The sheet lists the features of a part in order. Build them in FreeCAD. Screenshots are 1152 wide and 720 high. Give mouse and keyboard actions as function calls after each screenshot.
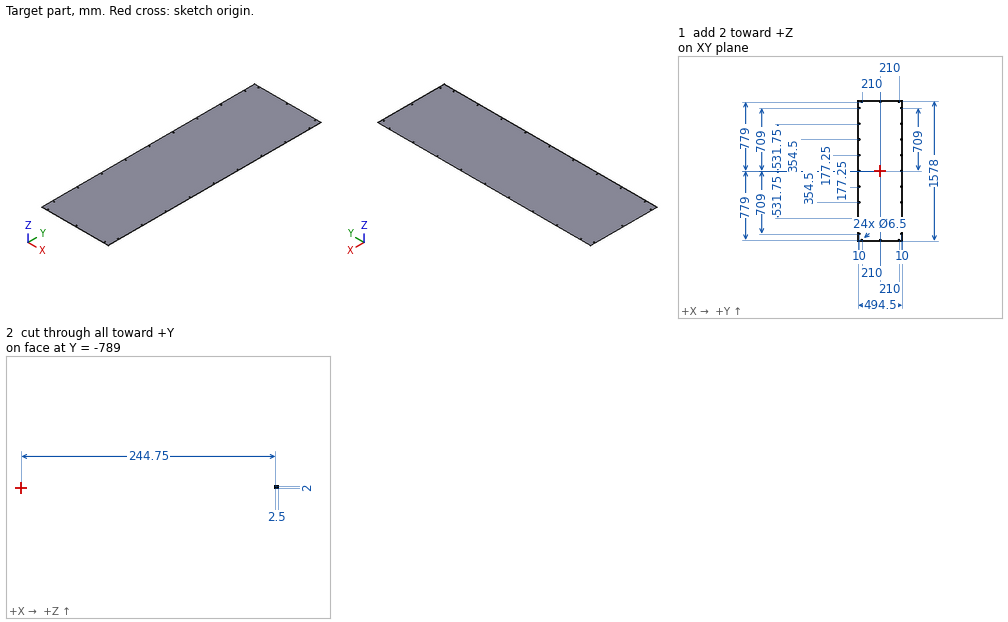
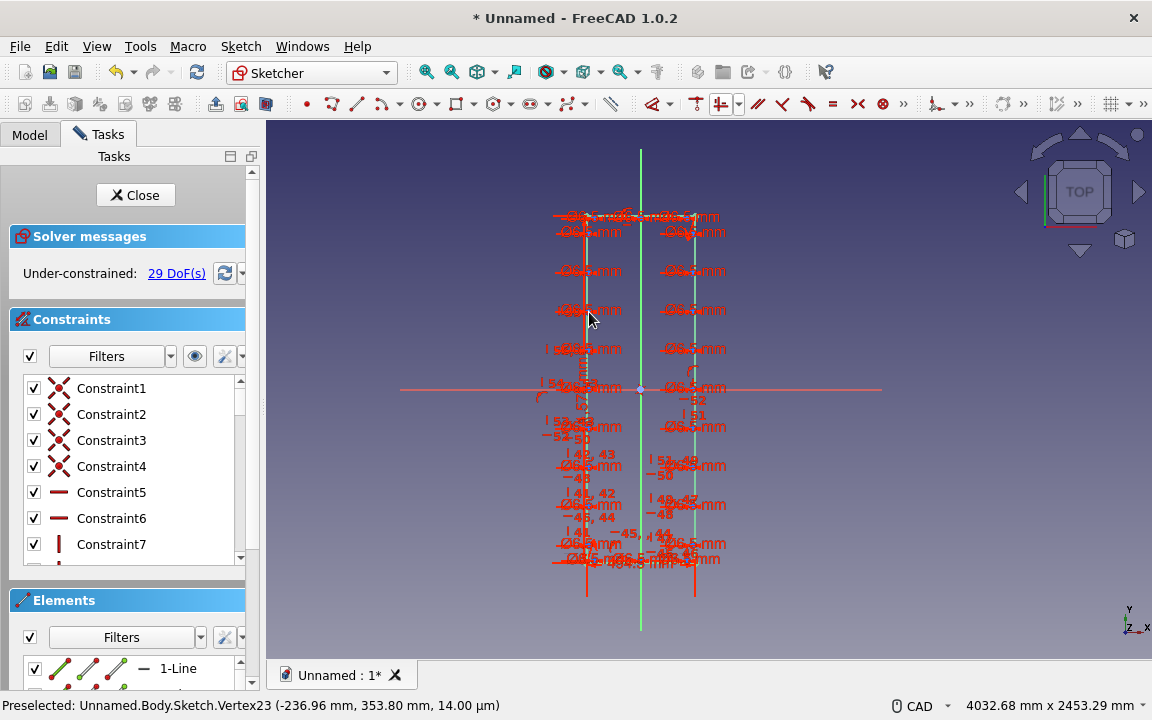
click(589, 312)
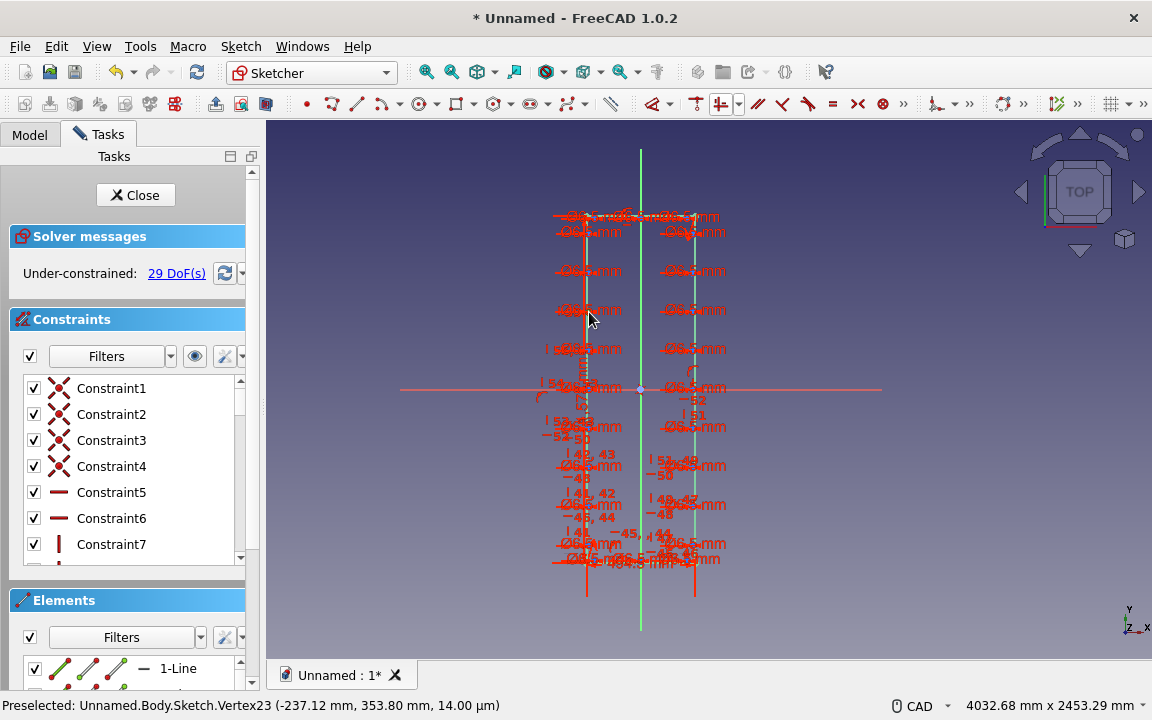
click(589, 273)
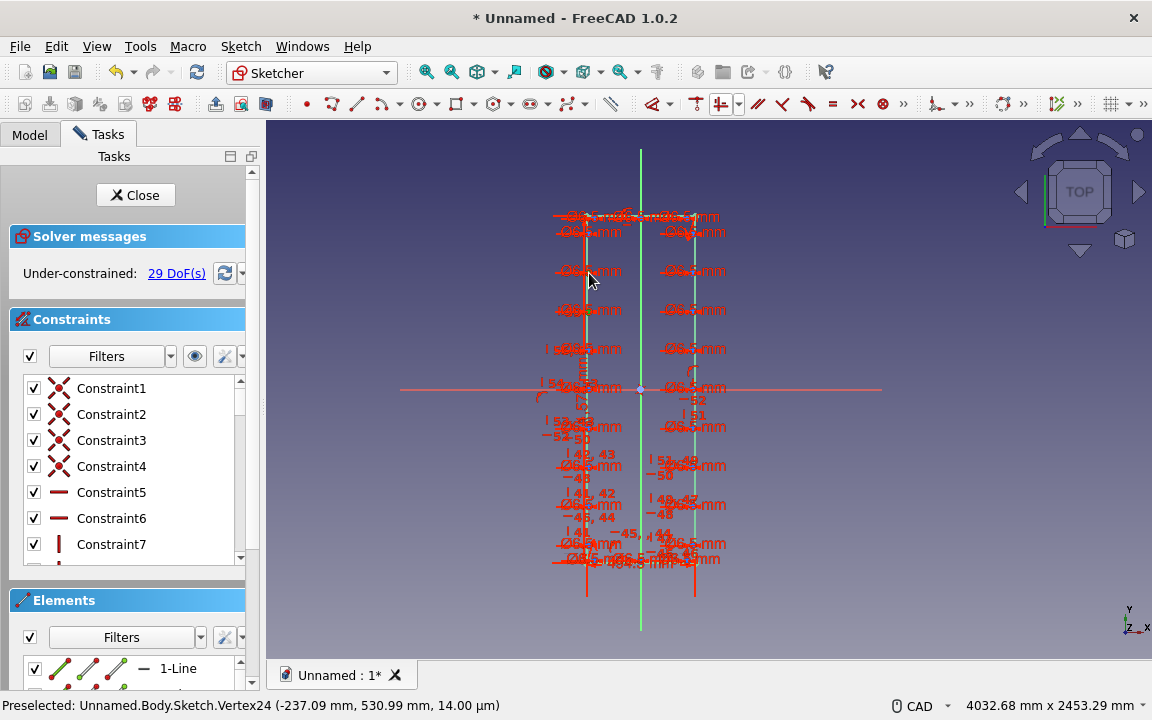
click(738, 104)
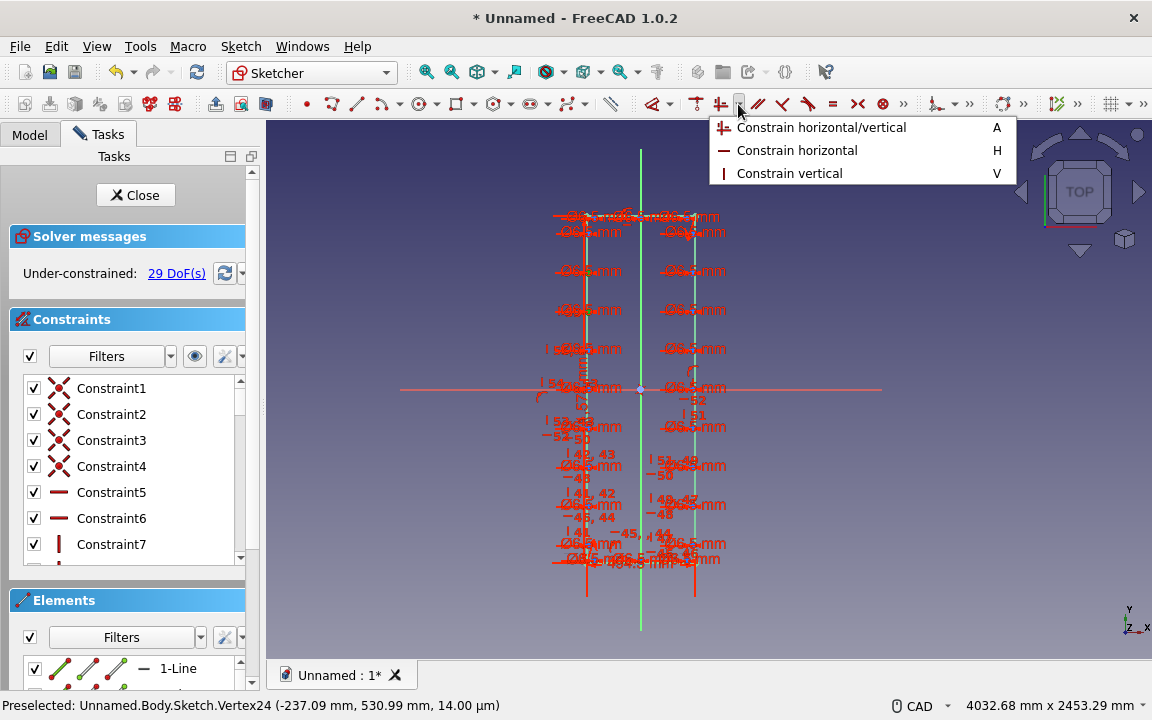
click(863, 174)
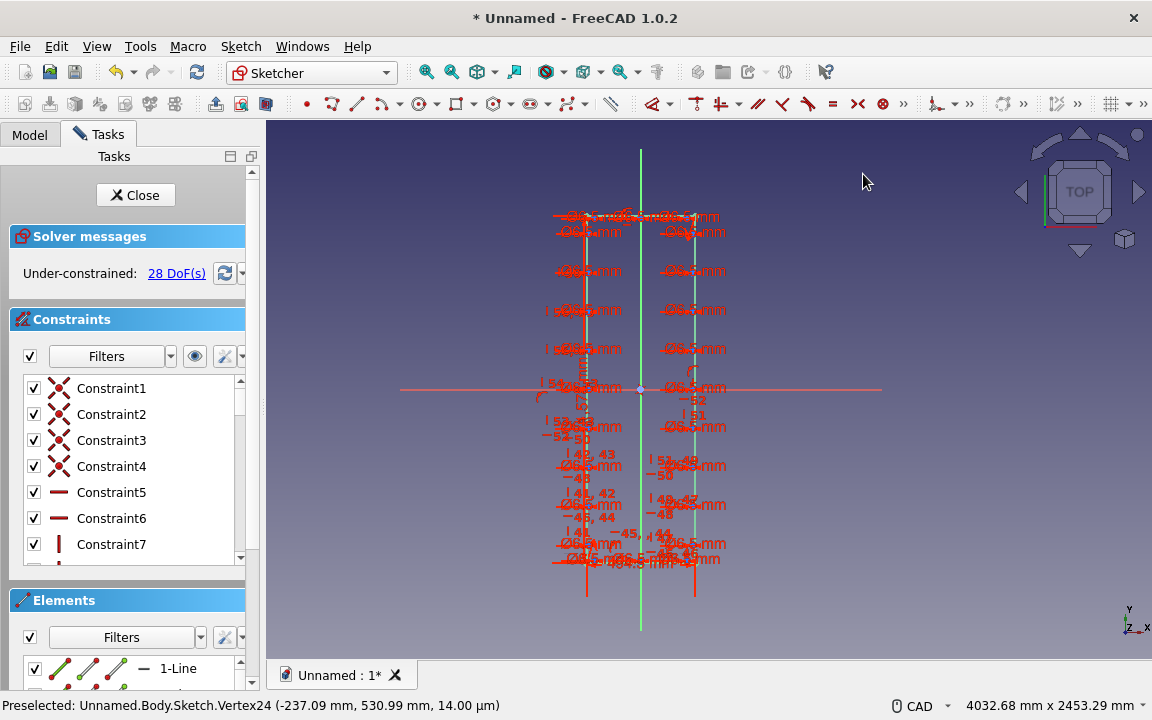
click(589, 273)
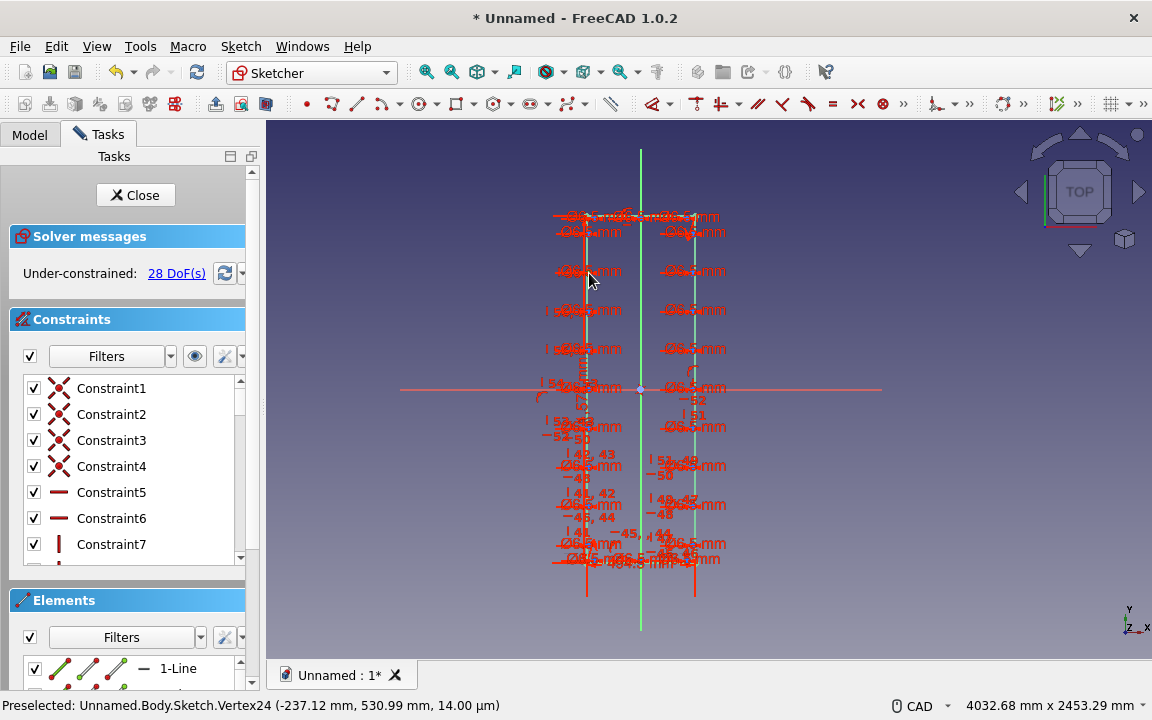
click(589, 234)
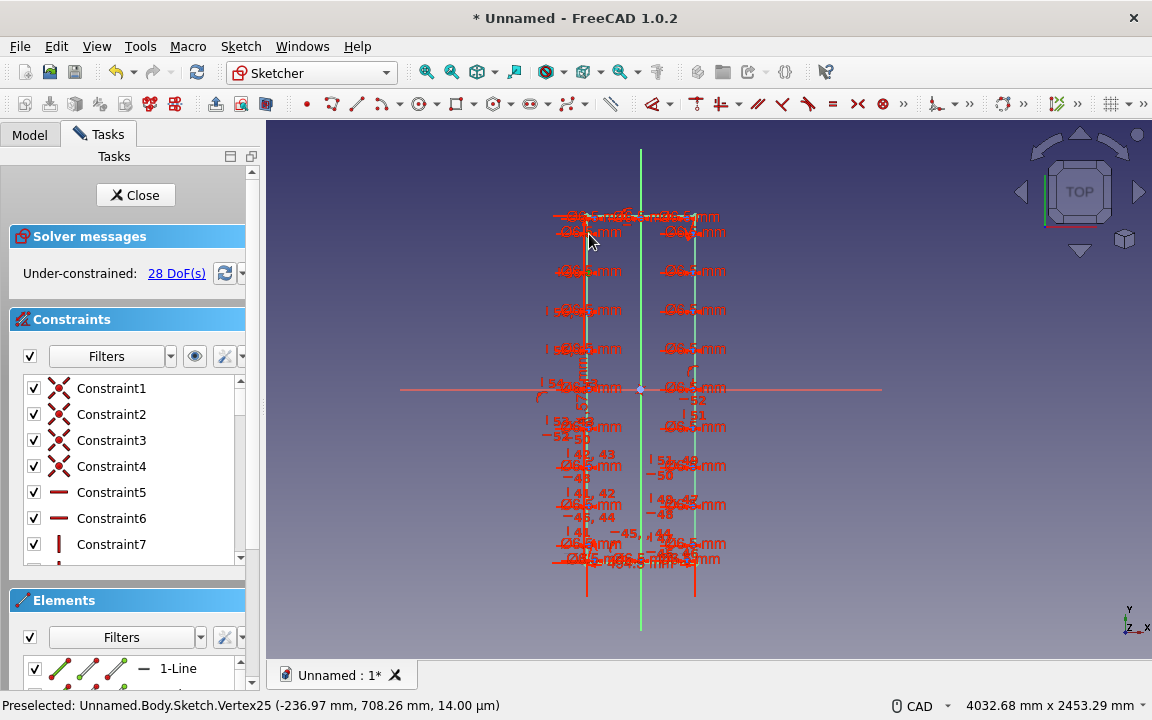
key(v)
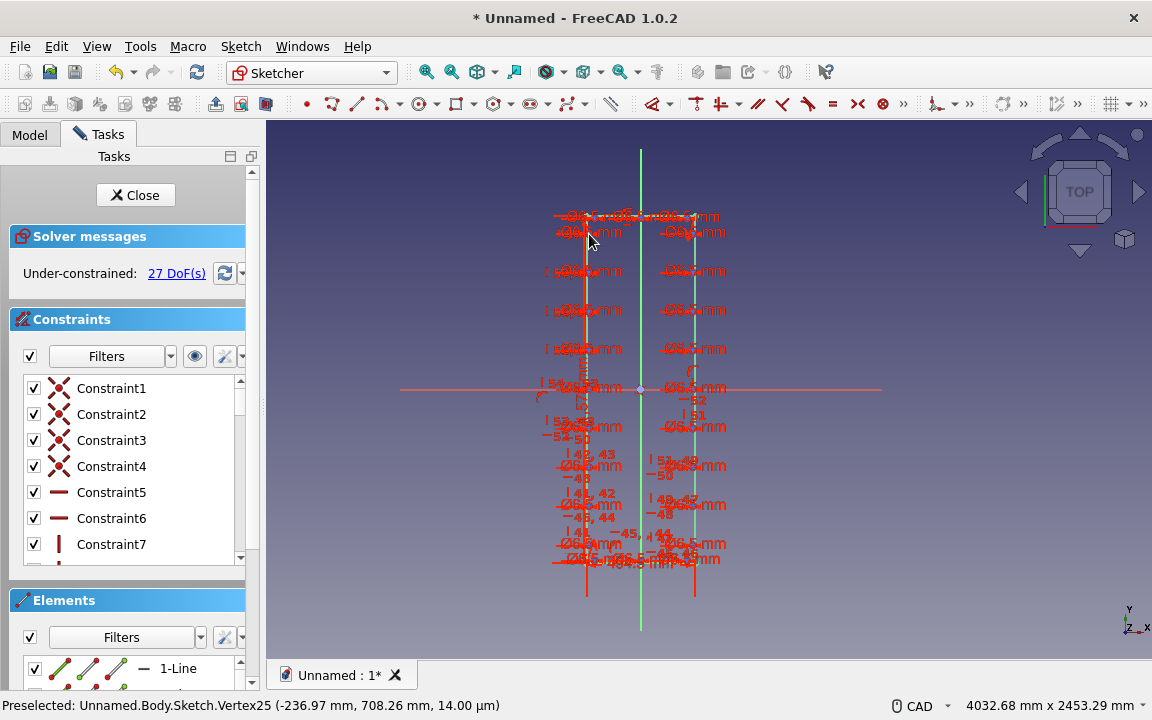
click(693, 429)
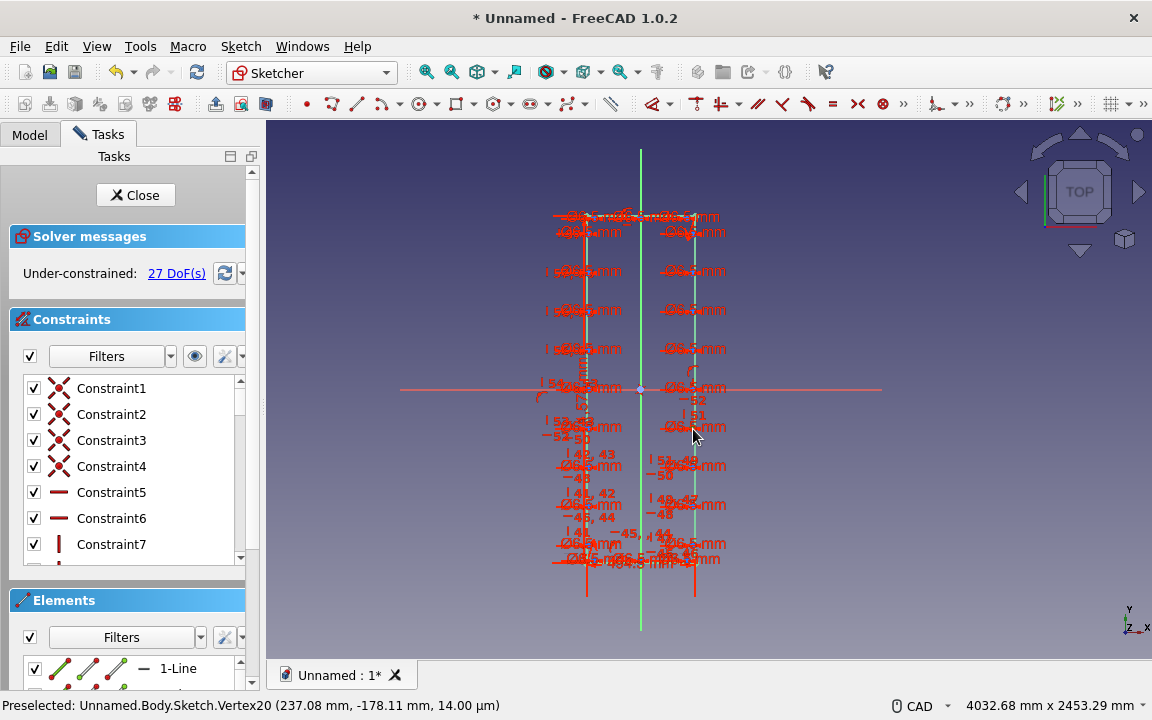
click(693, 390)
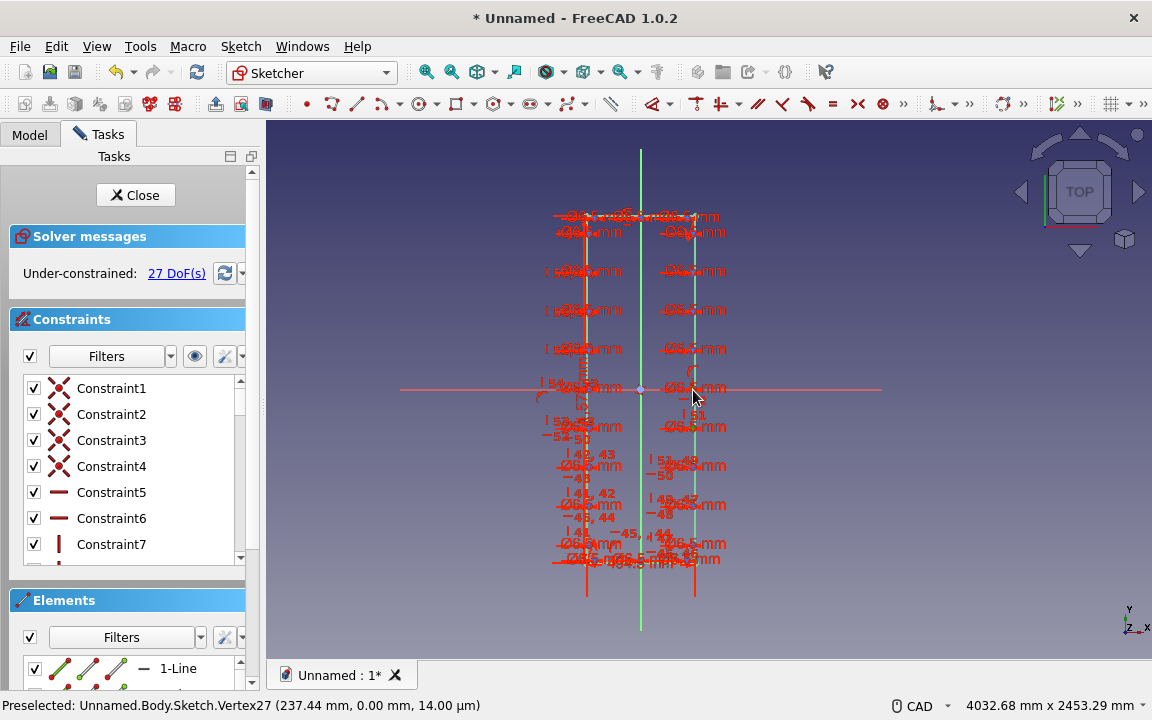
key(v)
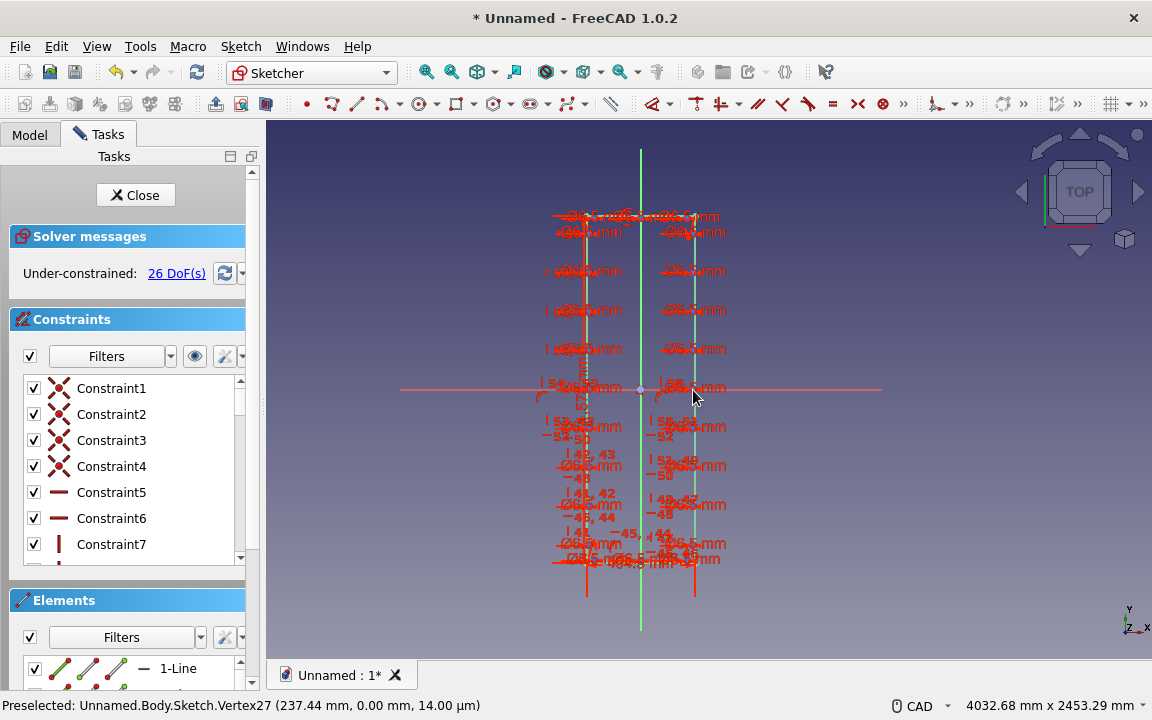
click(693, 390)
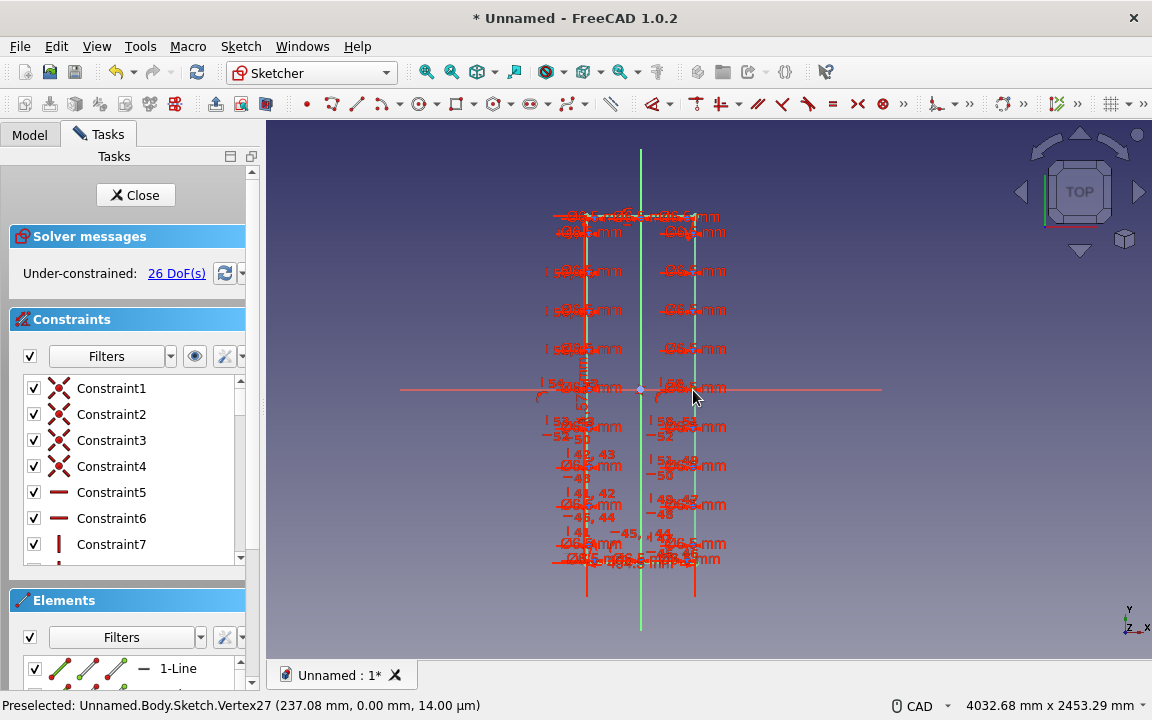
click(693, 351)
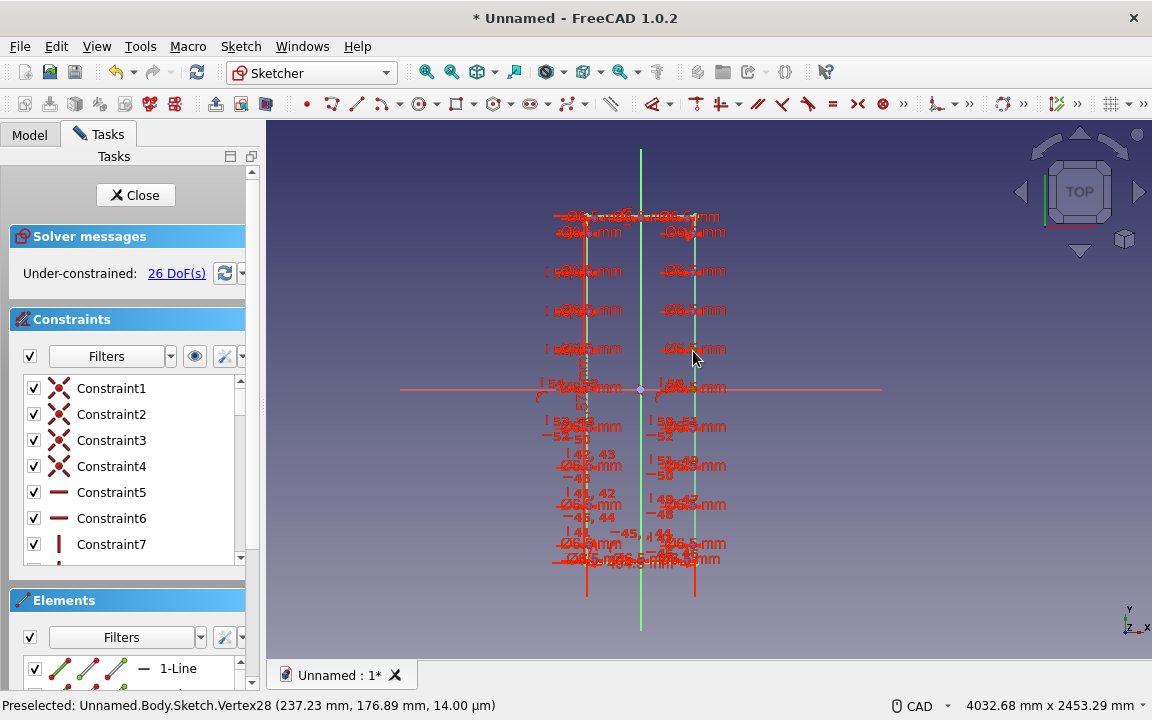
click(738, 104)